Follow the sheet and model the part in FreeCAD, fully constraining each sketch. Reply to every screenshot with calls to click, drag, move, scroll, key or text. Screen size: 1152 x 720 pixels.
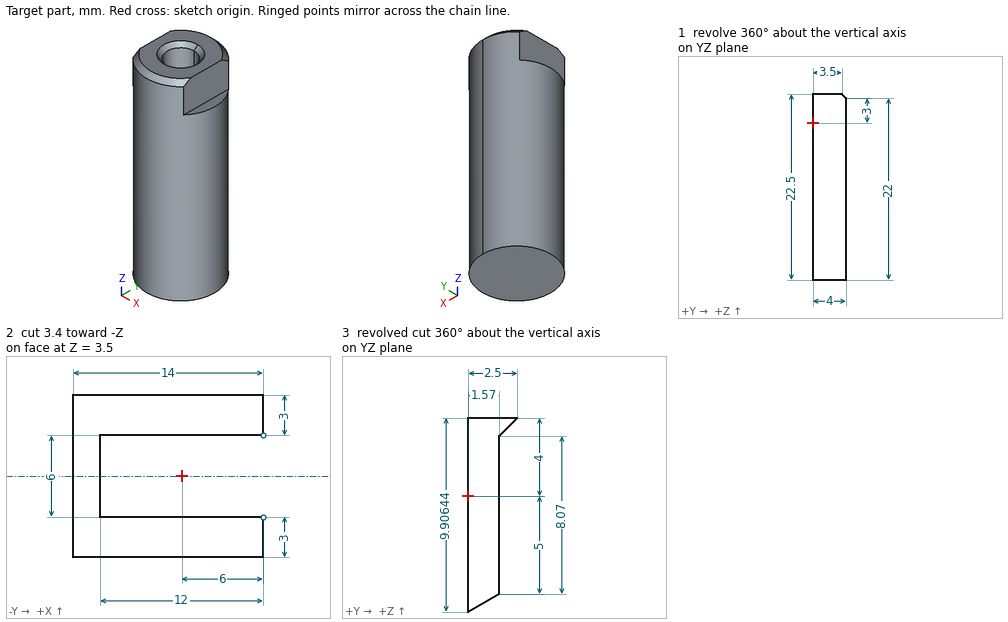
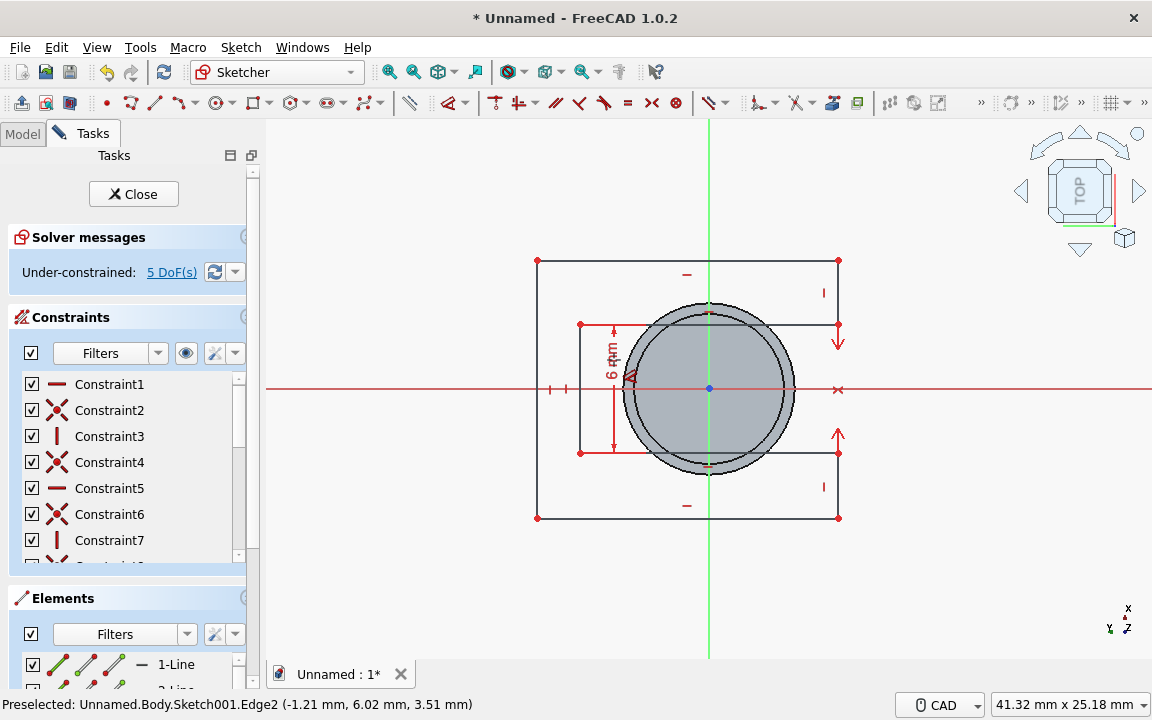
click(838, 306)
click(872, 293)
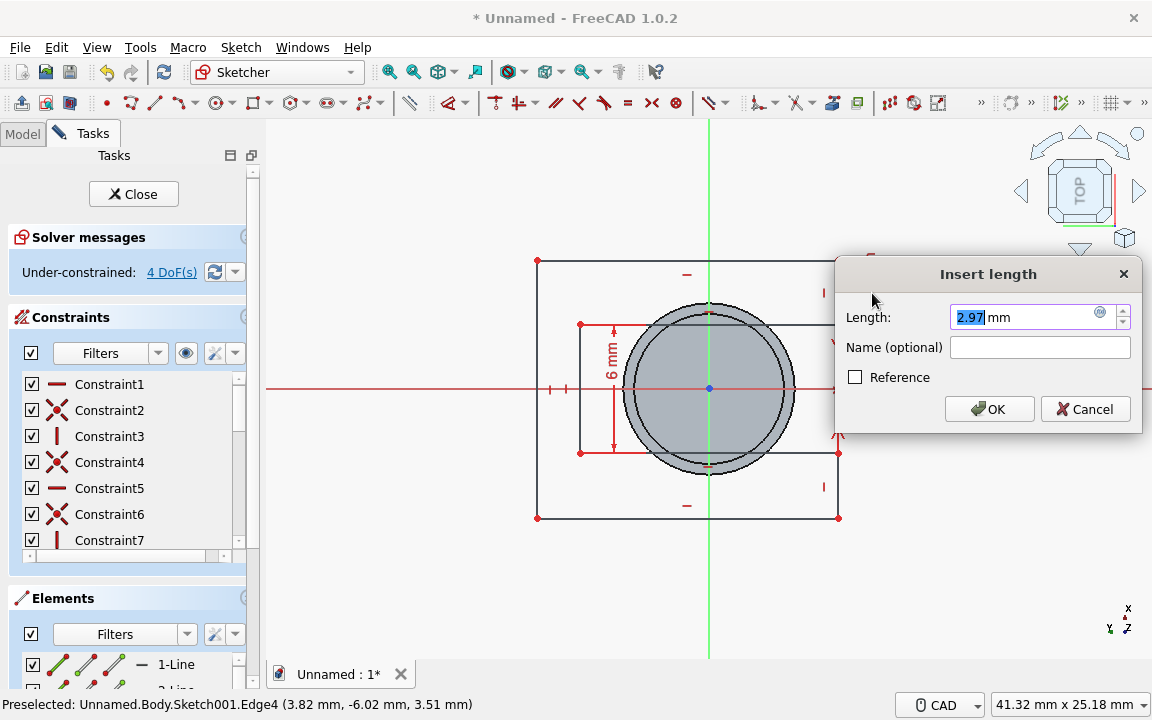
text(3)
key(Return)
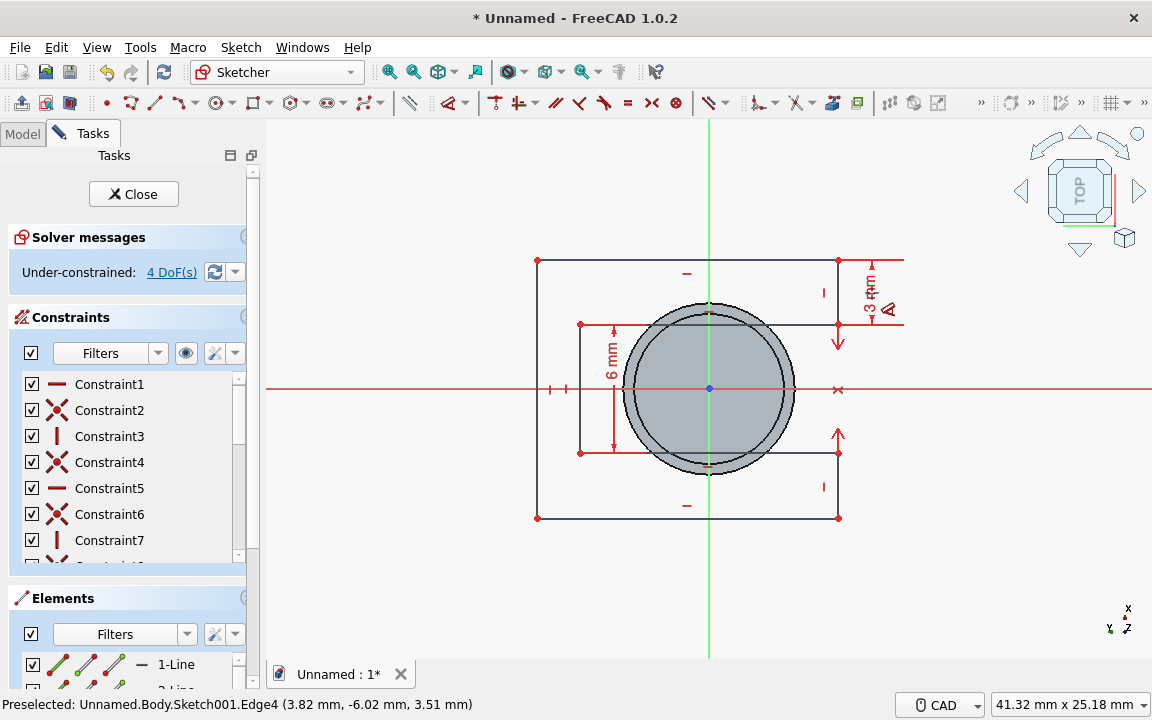
click(838, 499)
click(872, 486)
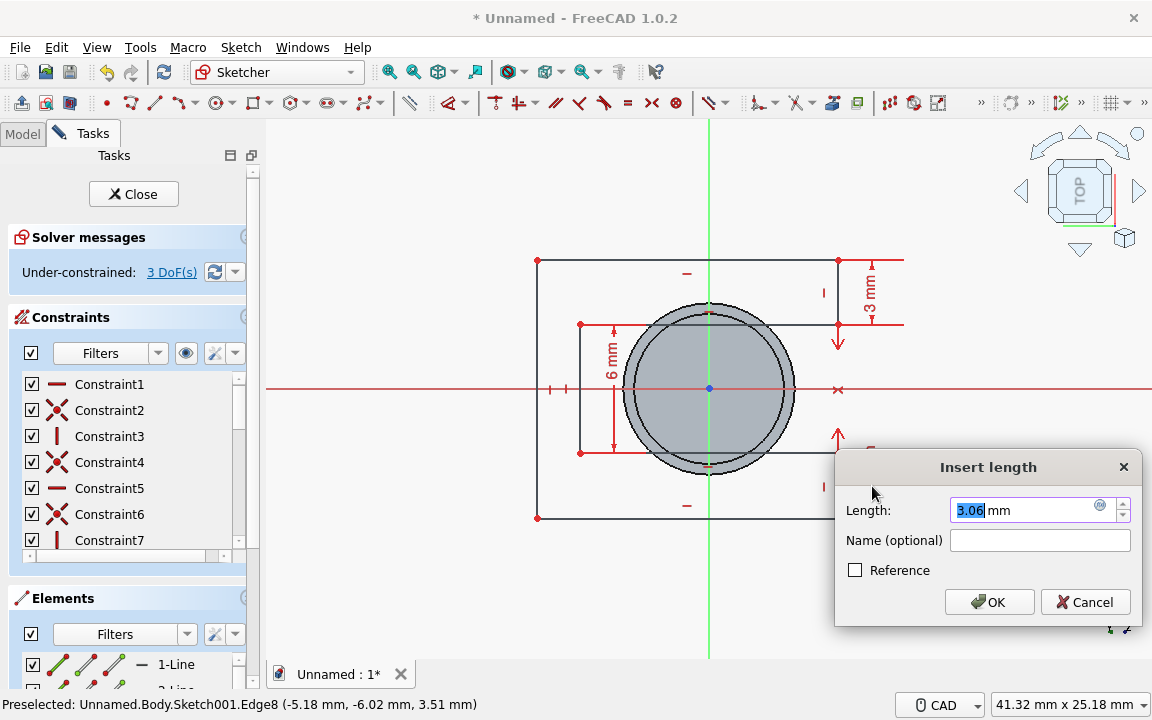
text(3)
key(Return)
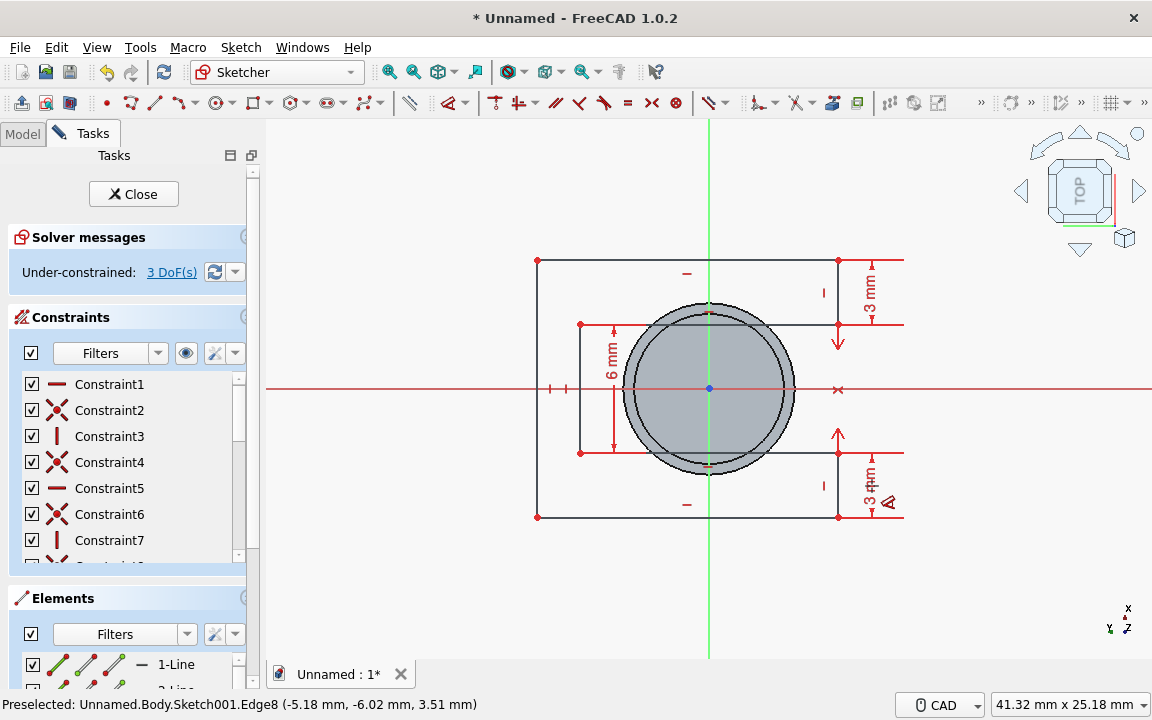
click(761, 453)
click(650, 487)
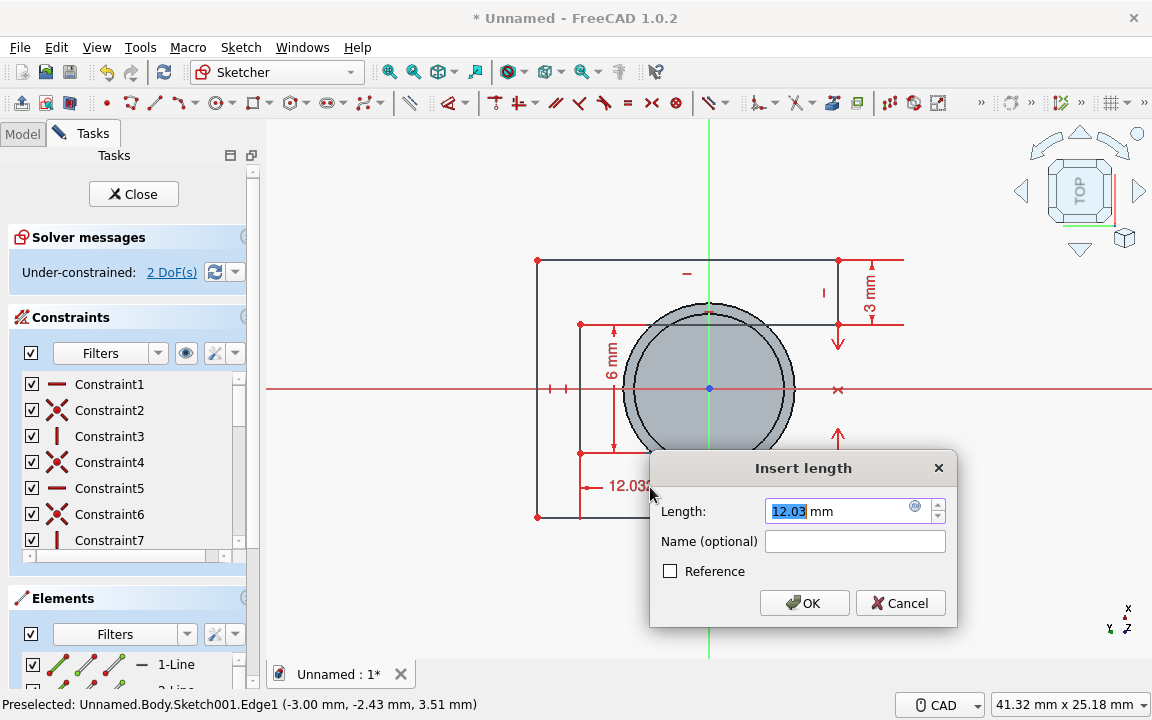
text(12)
key(Return)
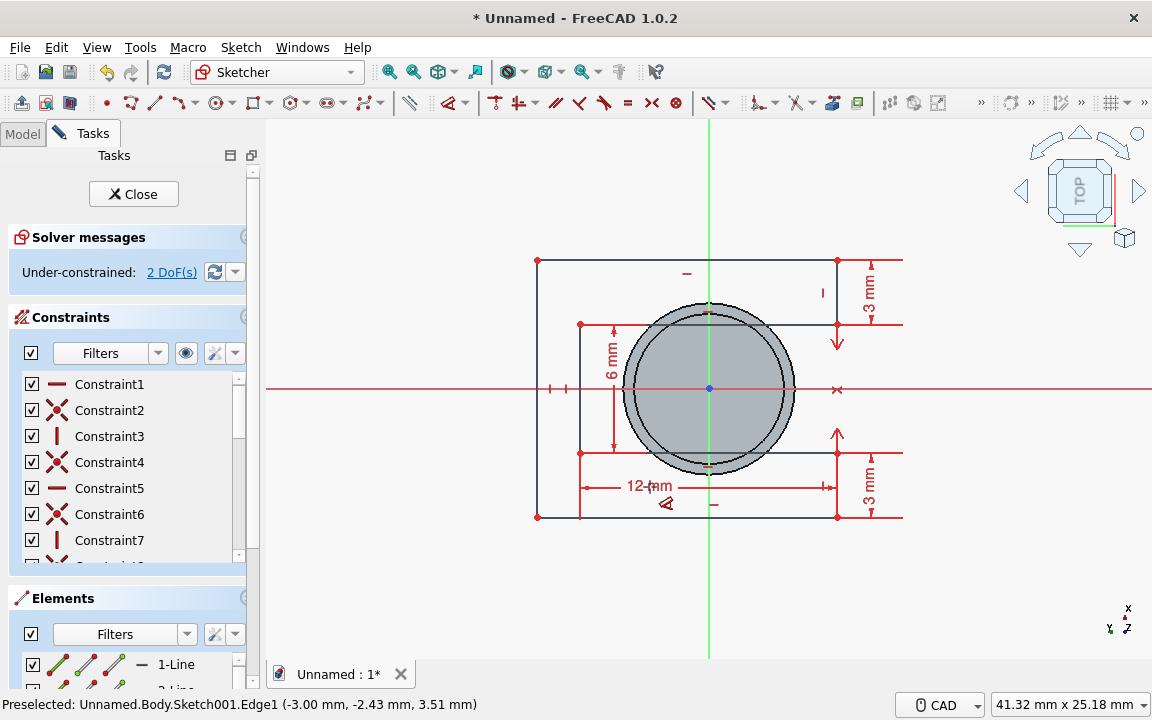
click(747, 260)
click(687, 226)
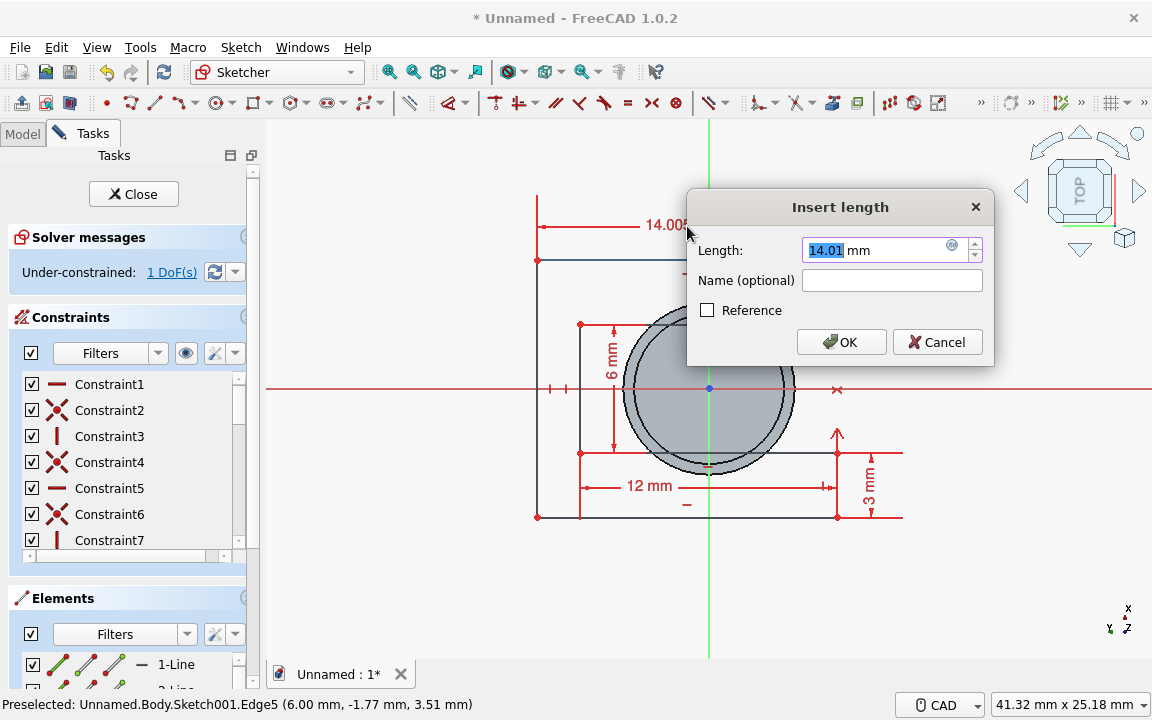
text(14)
key(Return)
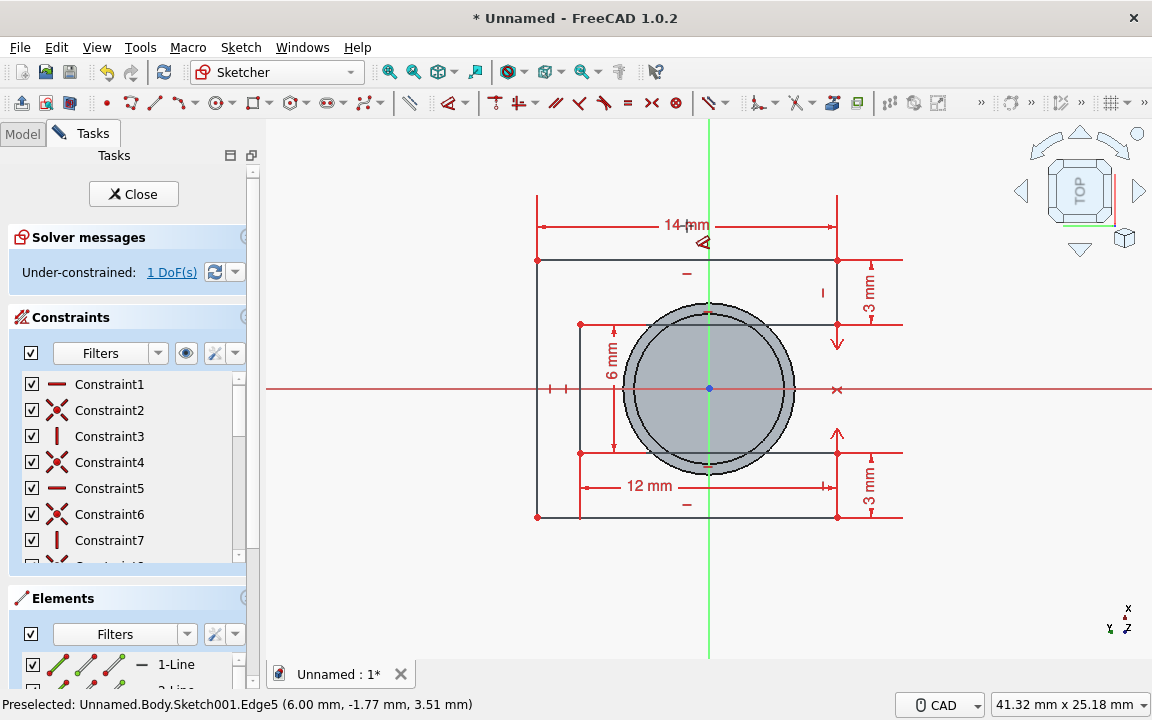
click(837, 453)
click(773, 487)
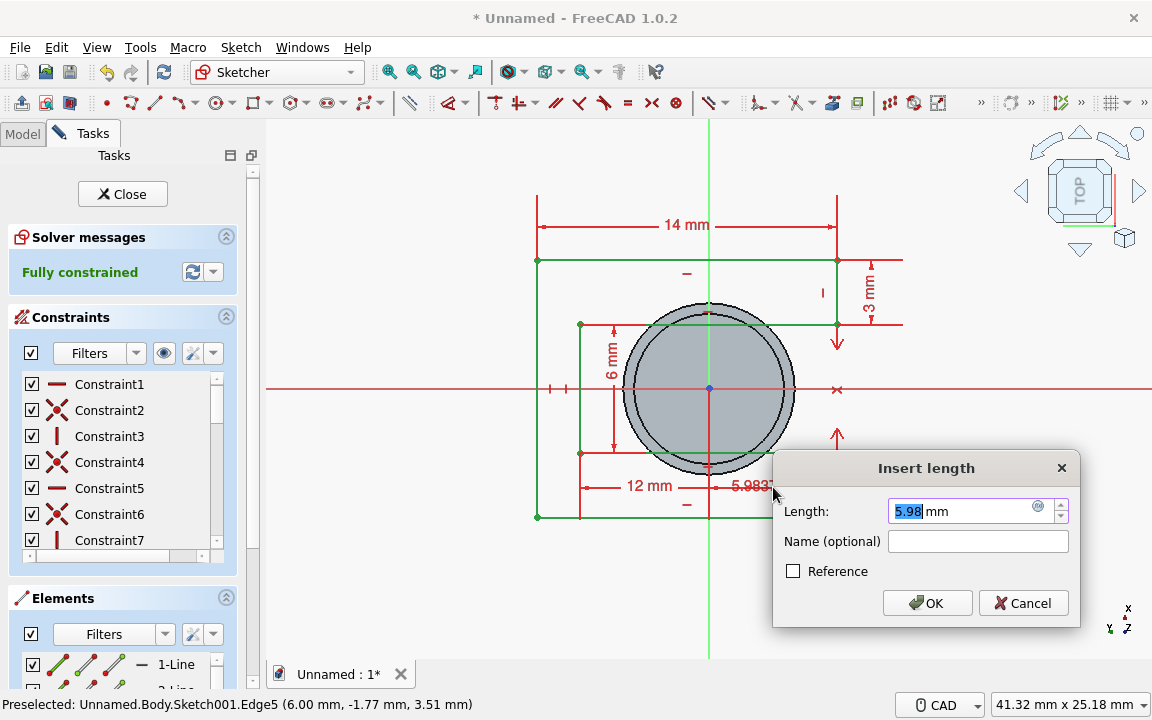
text(6)
key(Return)
key(Escape)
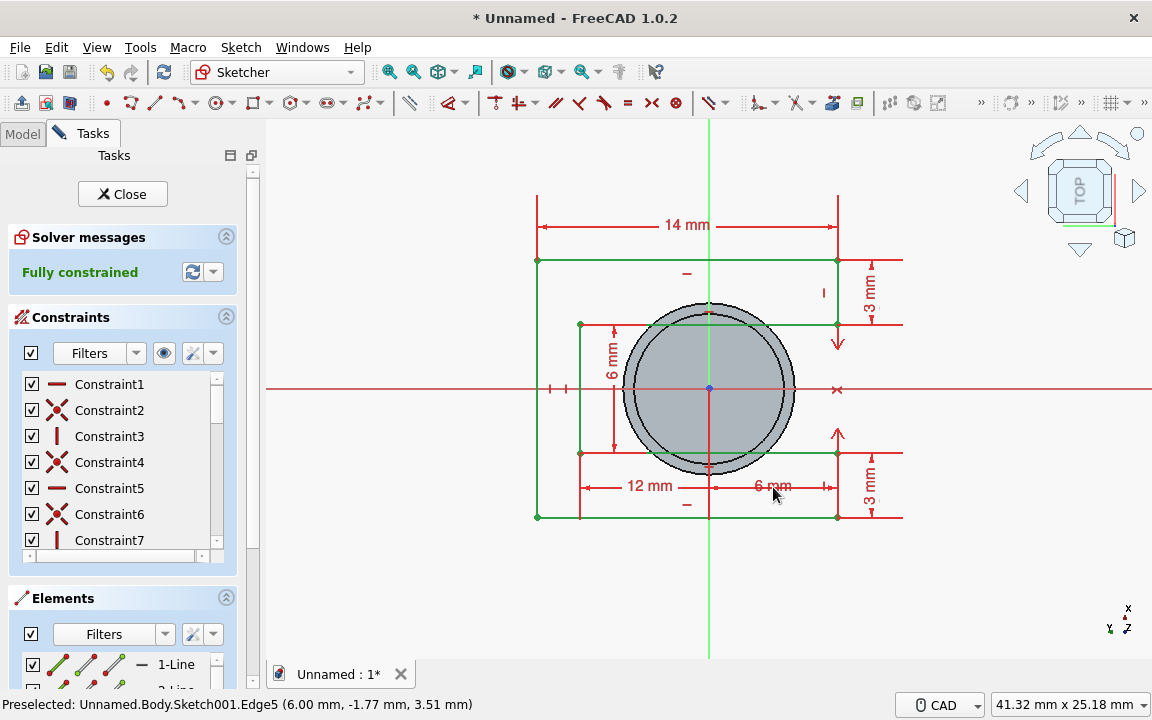
click(123, 194)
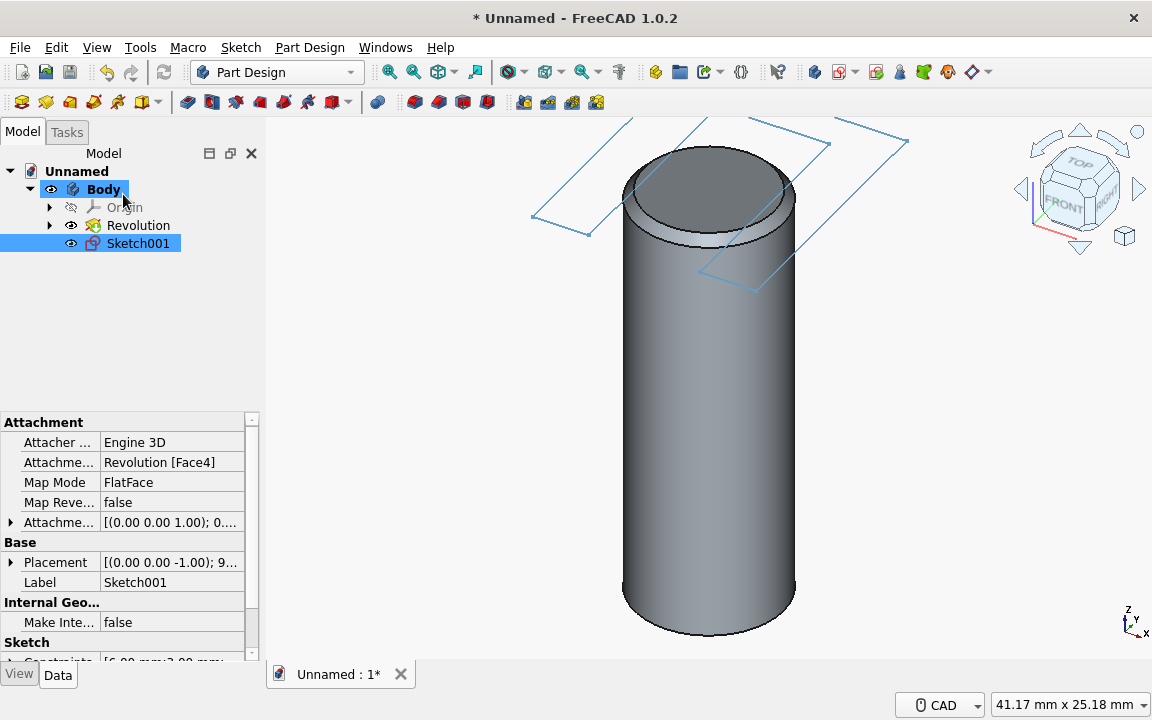
click(188, 102)